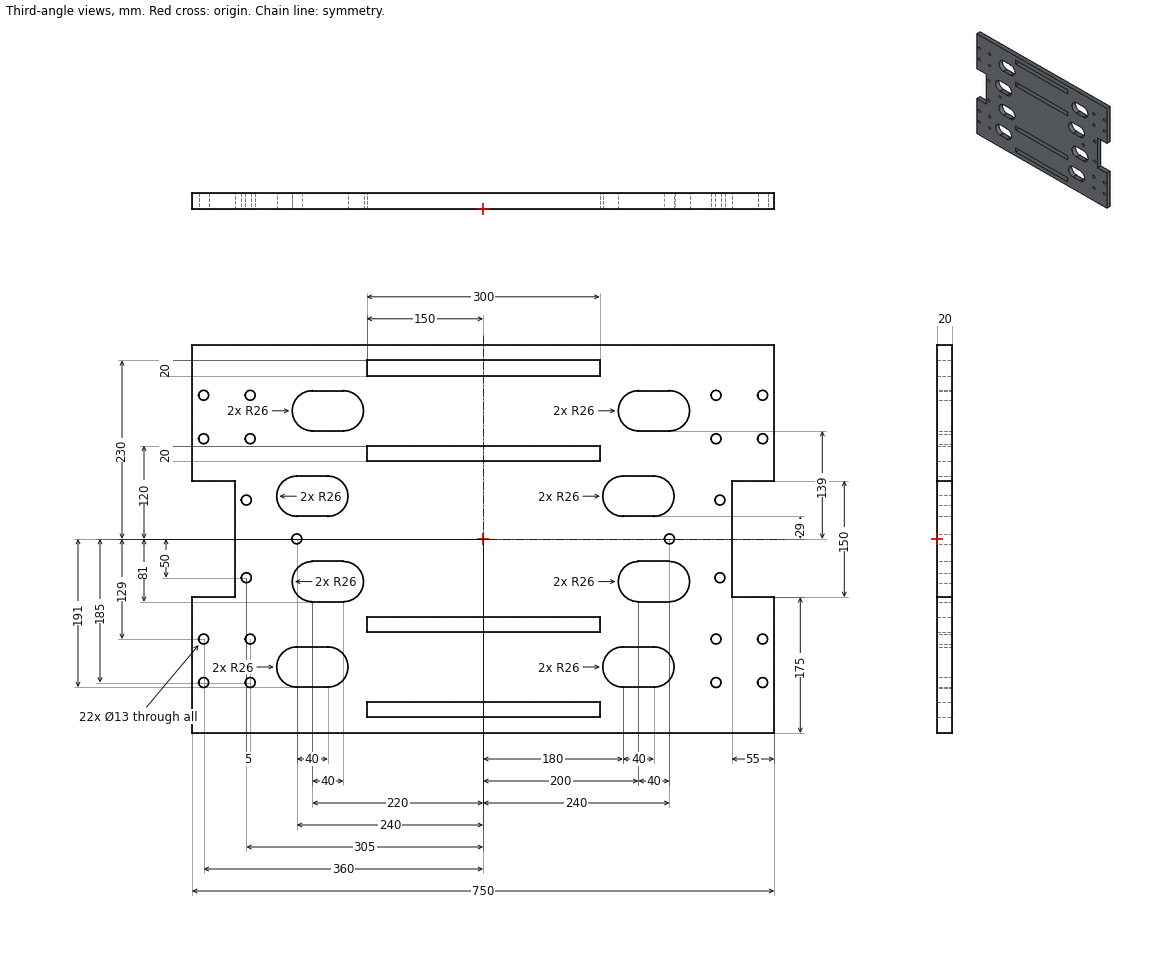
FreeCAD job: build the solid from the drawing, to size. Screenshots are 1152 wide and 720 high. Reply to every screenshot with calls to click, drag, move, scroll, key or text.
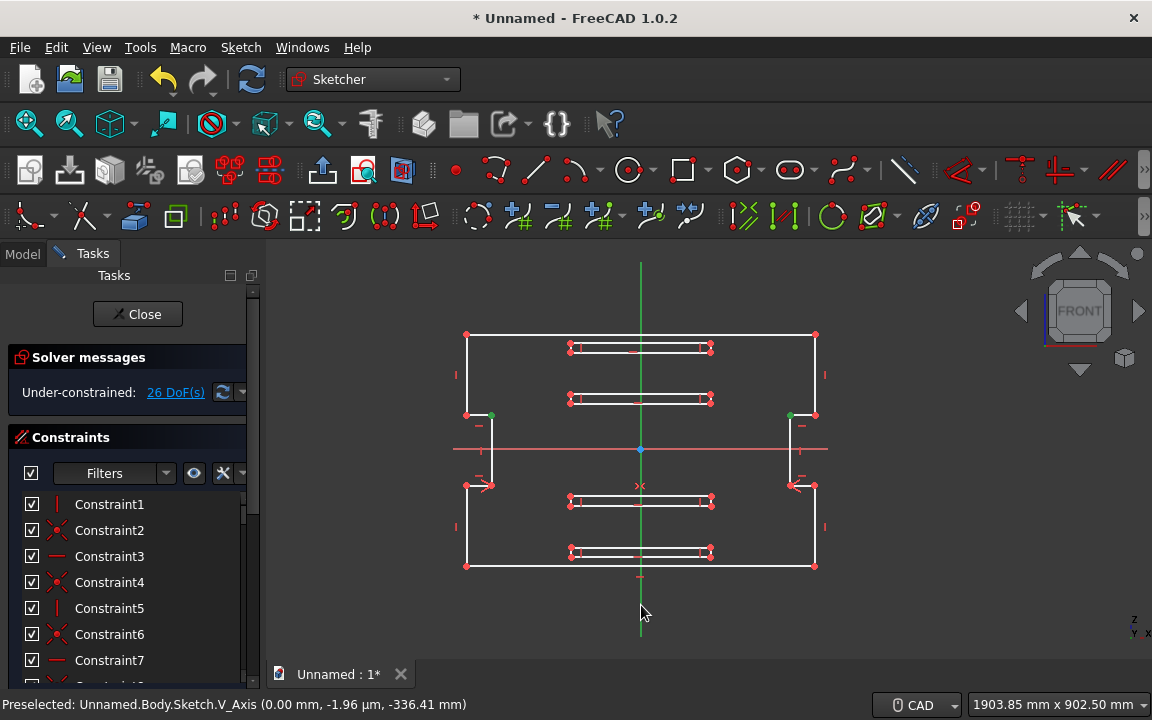
key(s)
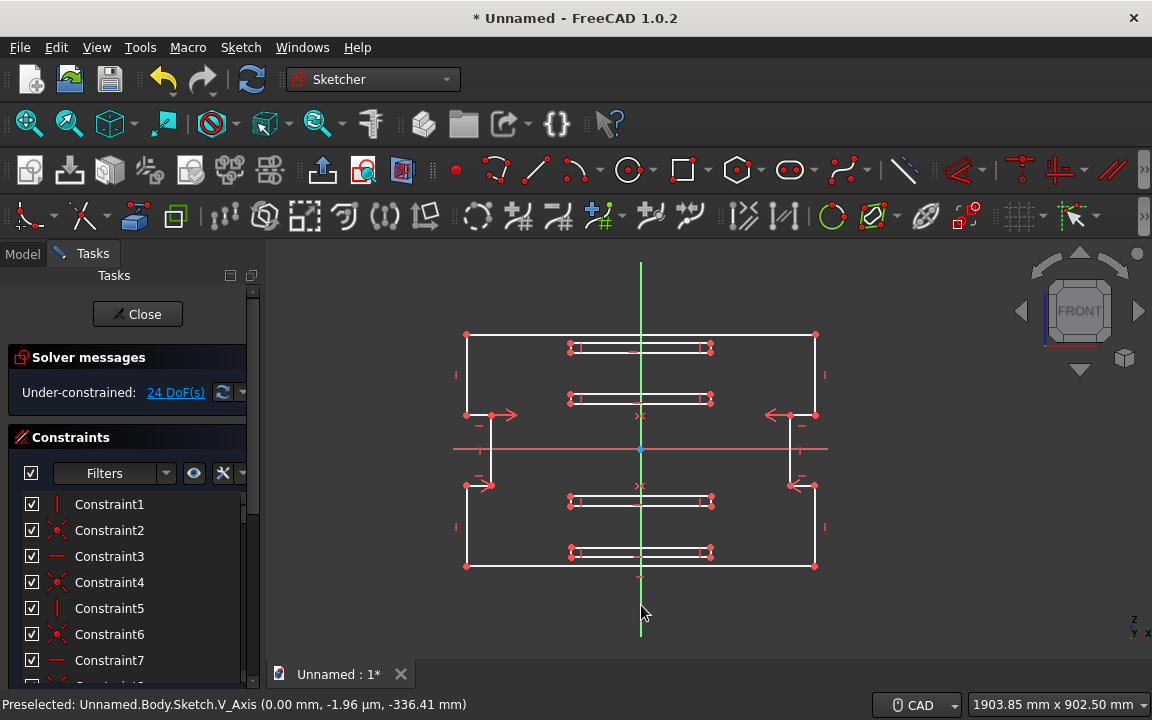
click(467, 486)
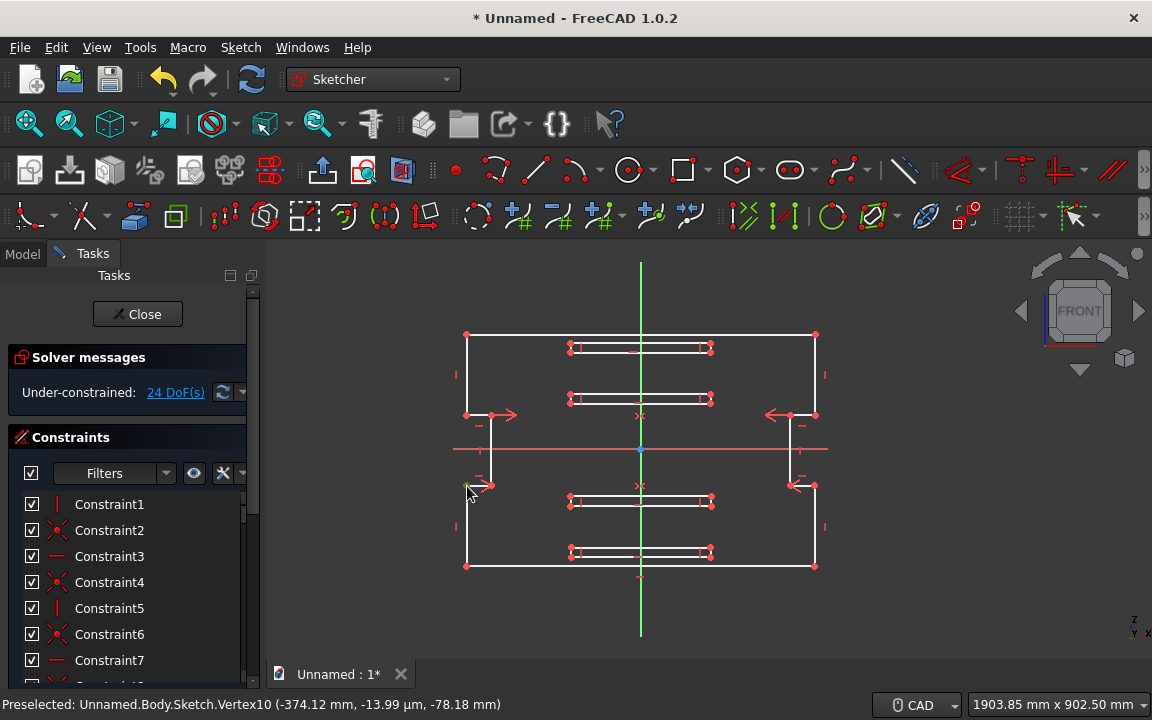
click(467, 415)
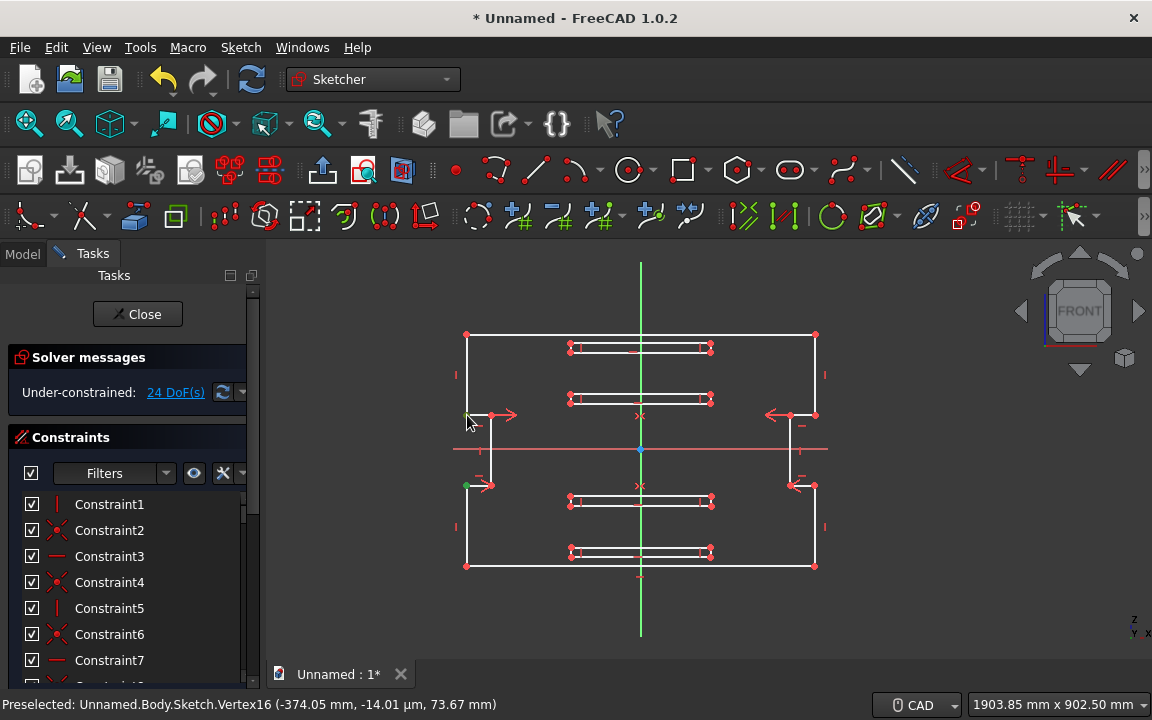
click(542, 449)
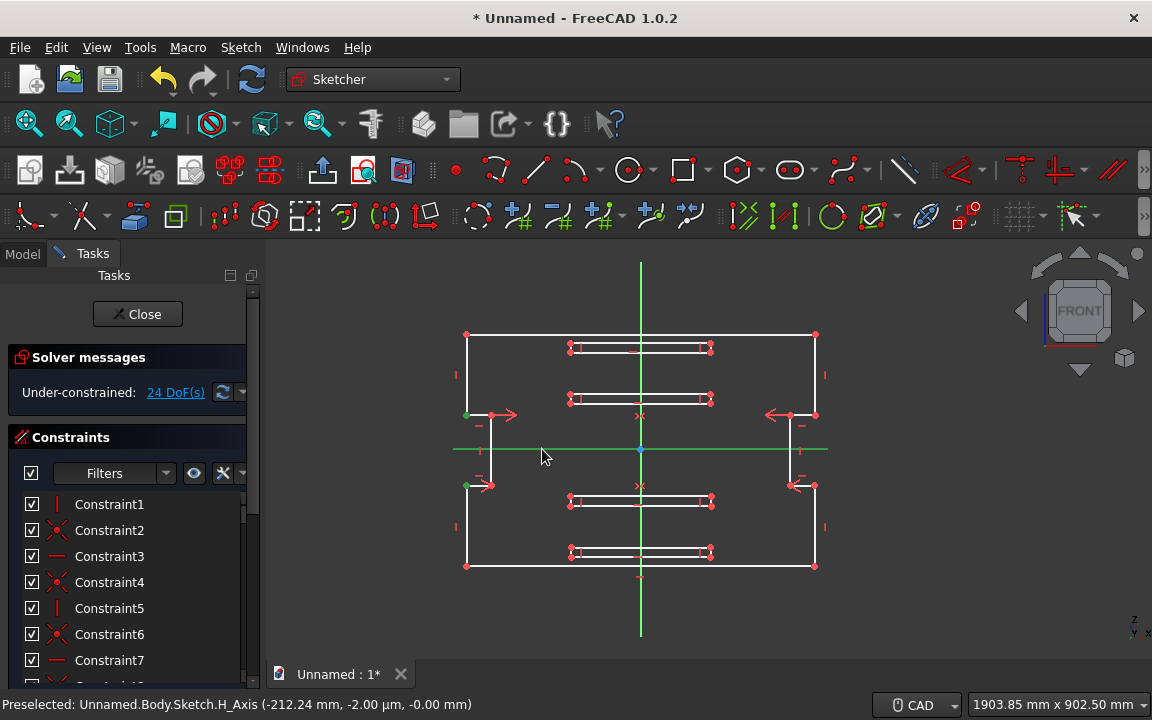
key(s)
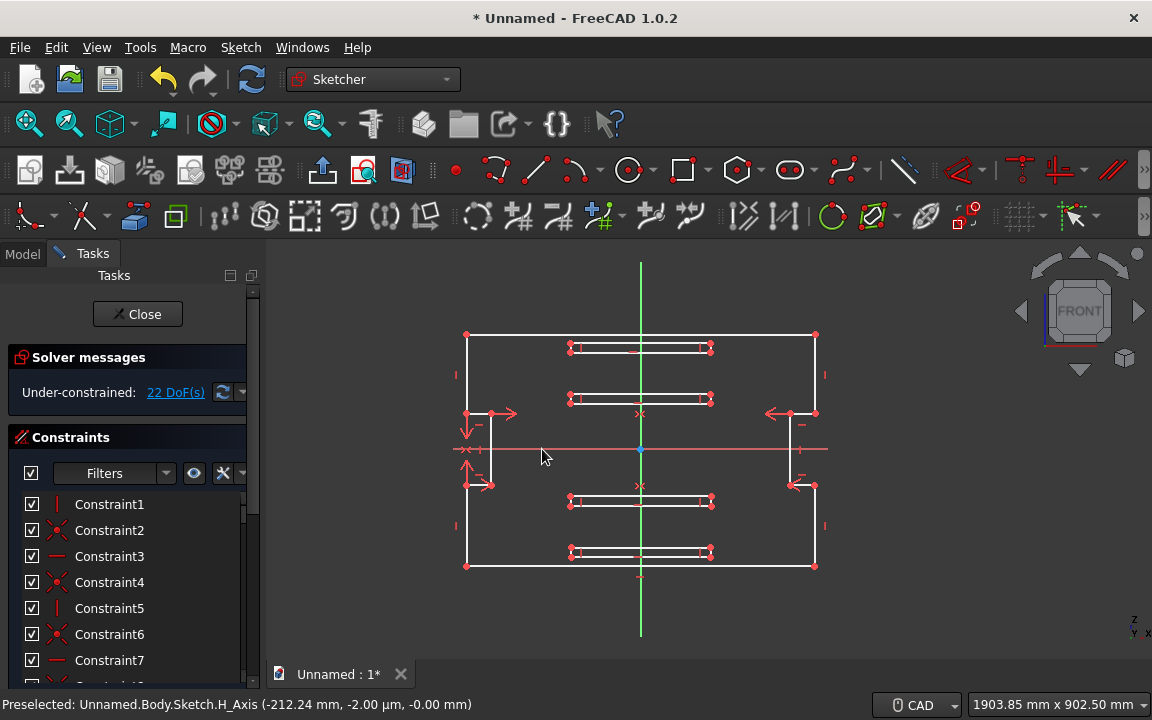
click(815, 566)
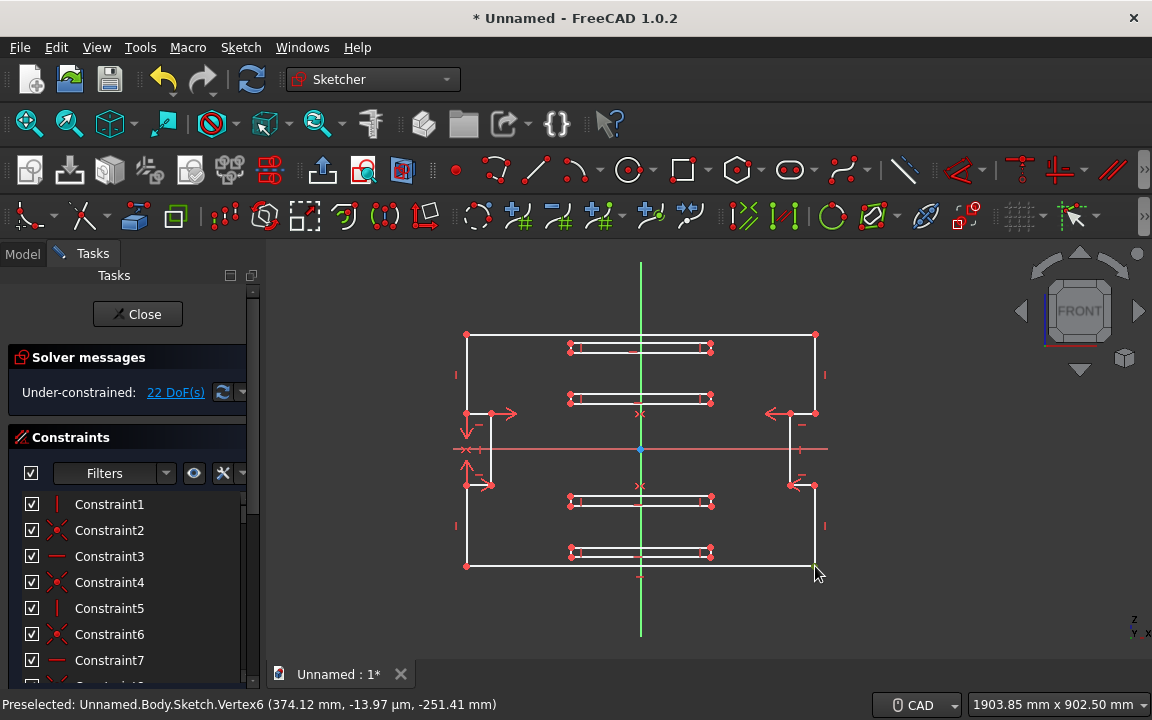
click(815, 335)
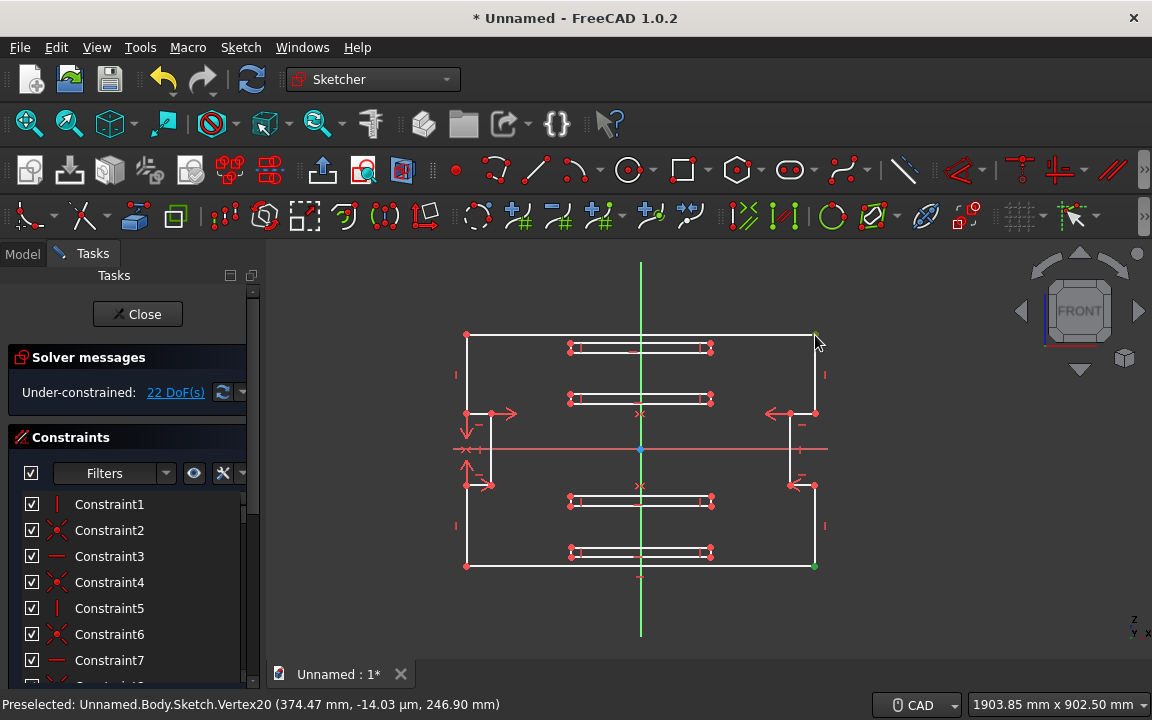
click(542, 449)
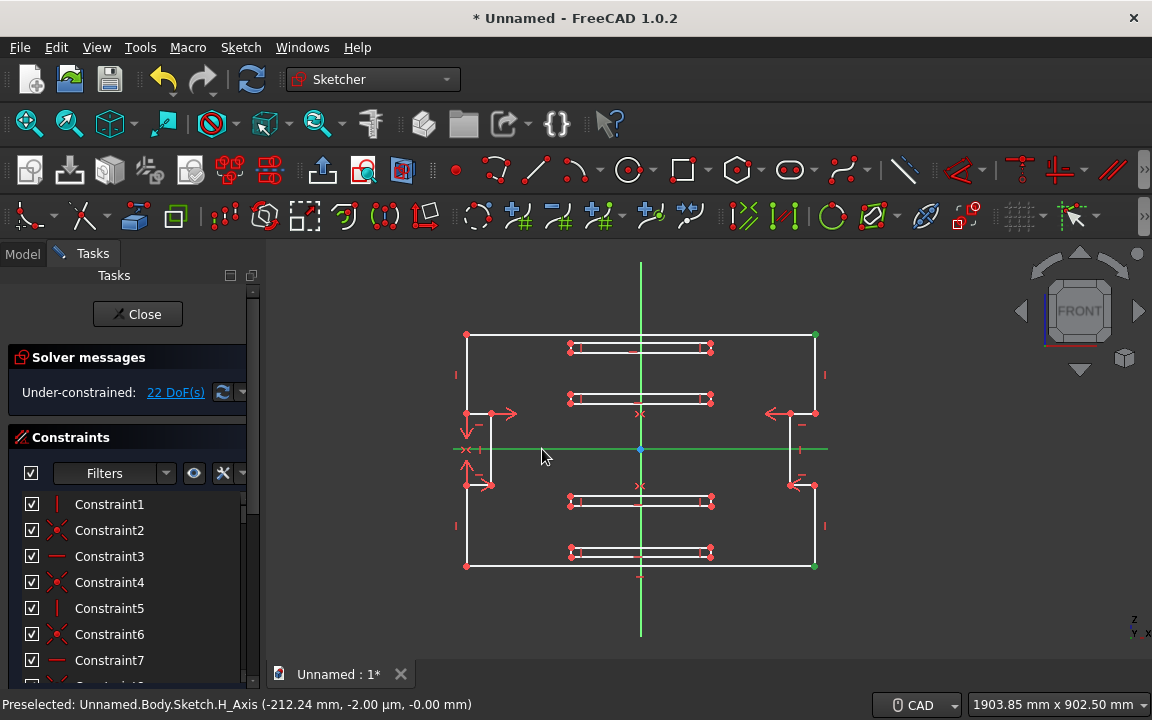
key(s)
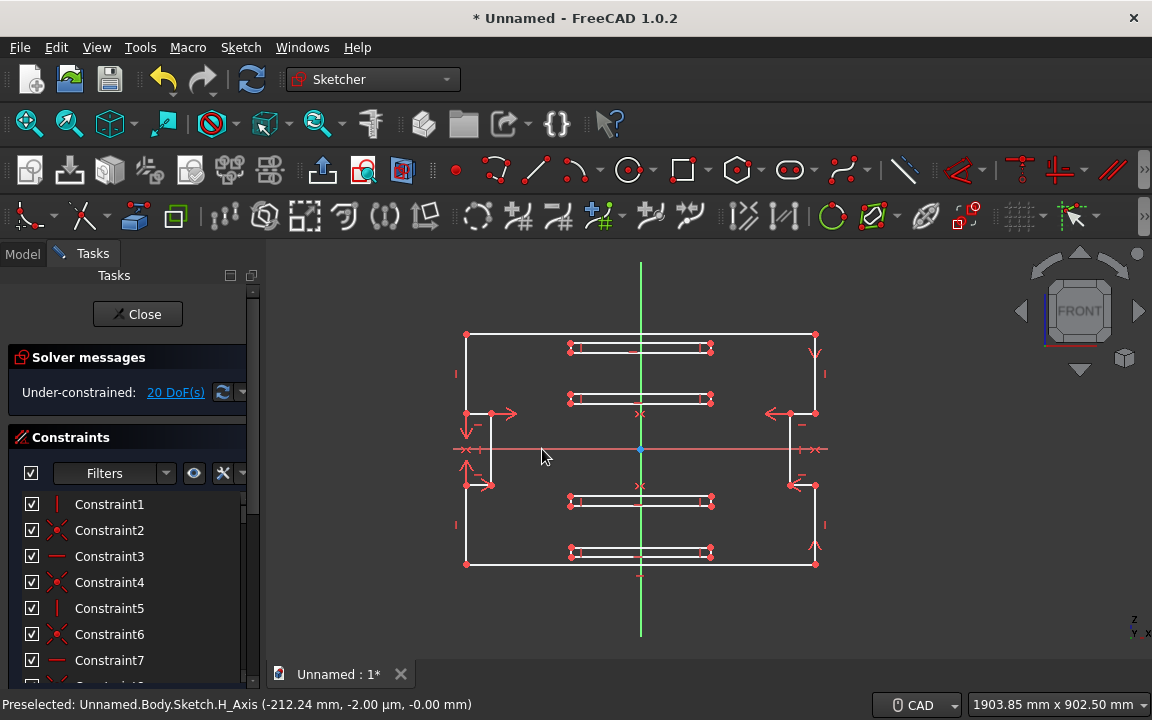
scroll(571, 404, up, 2)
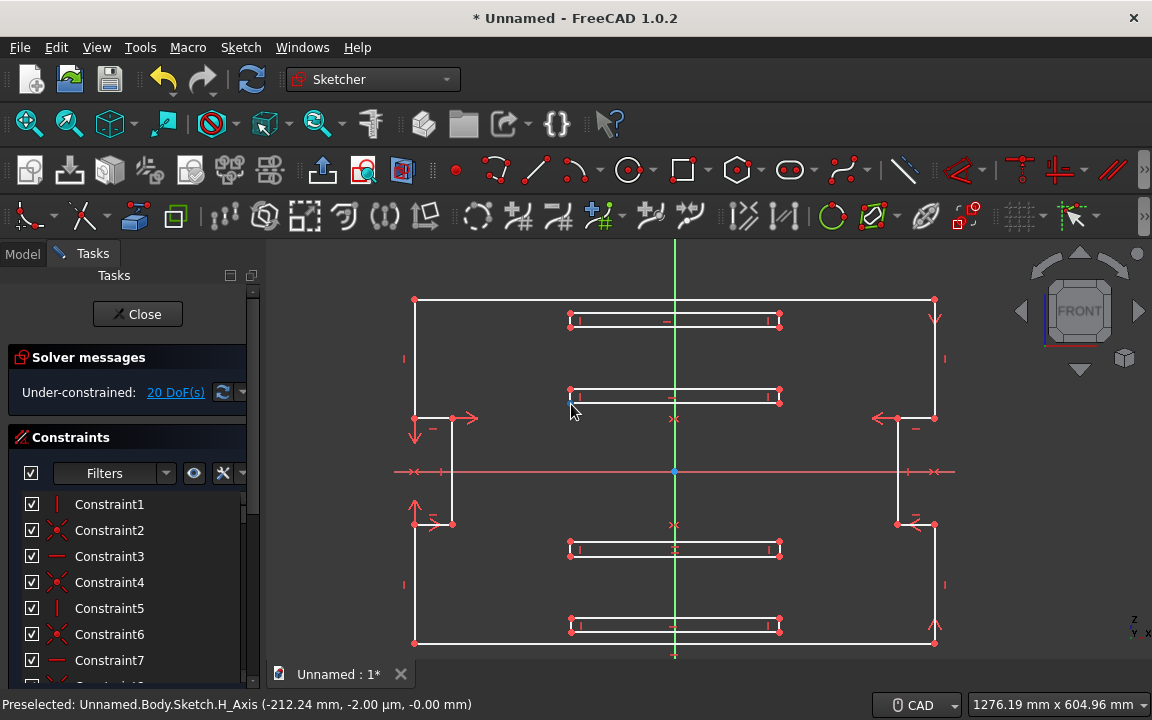
click(570, 403)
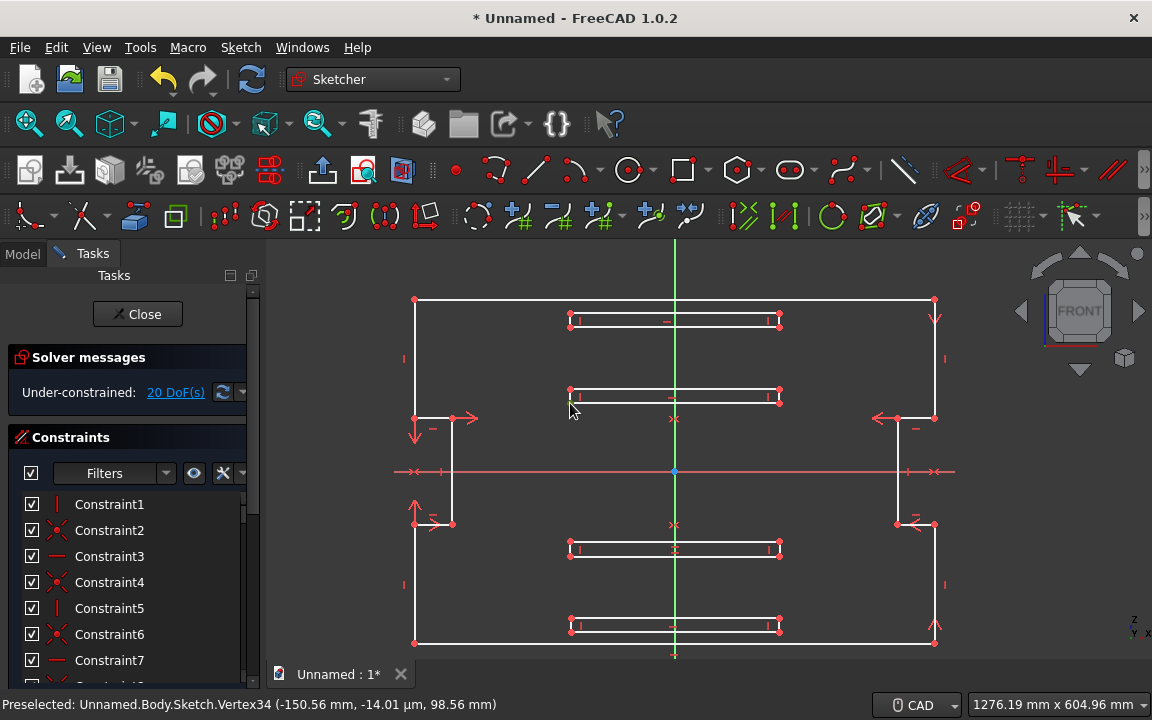
click(570, 542)